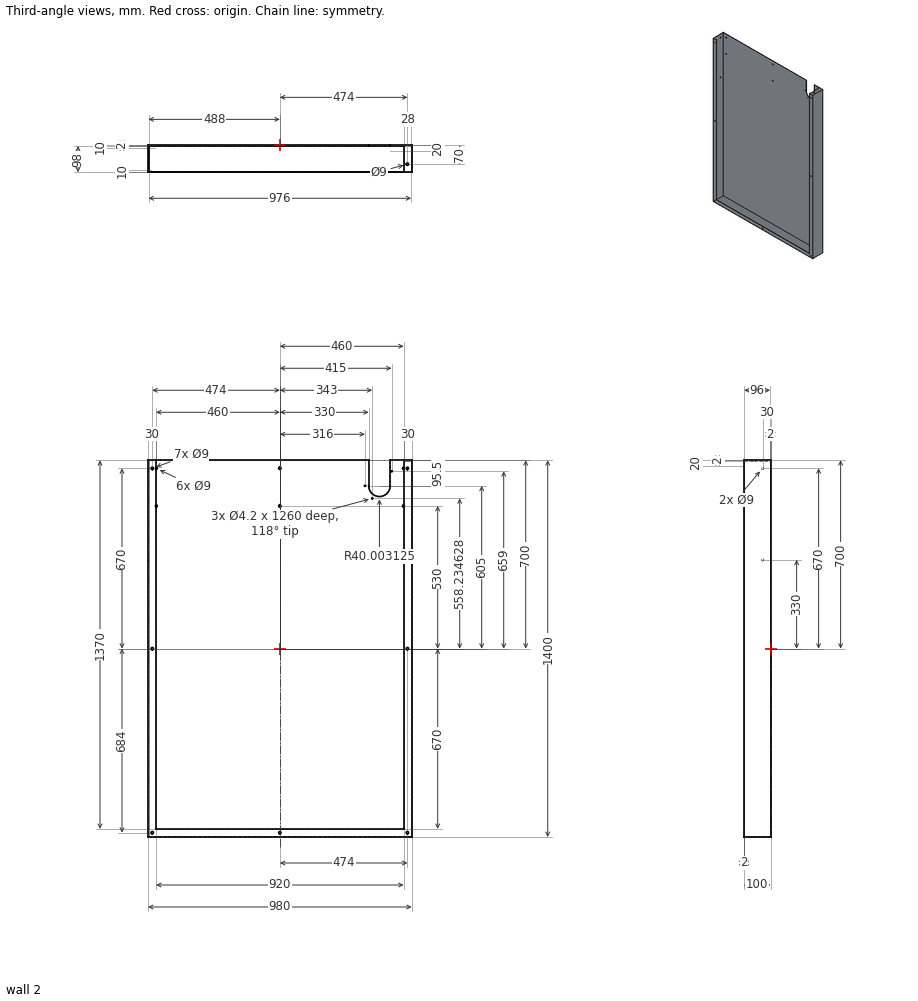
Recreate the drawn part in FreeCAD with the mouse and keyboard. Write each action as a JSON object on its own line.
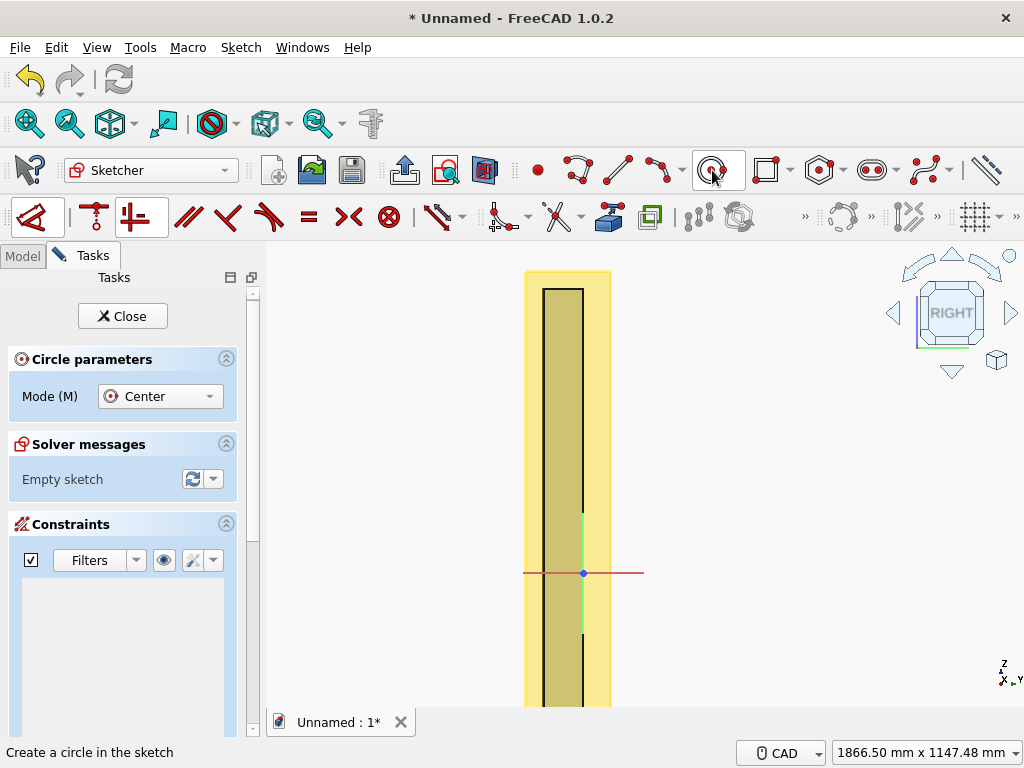
{"action": "scroll", "coordinate": [571, 301], "scroll_direction": "up", "scroll_amount": 13}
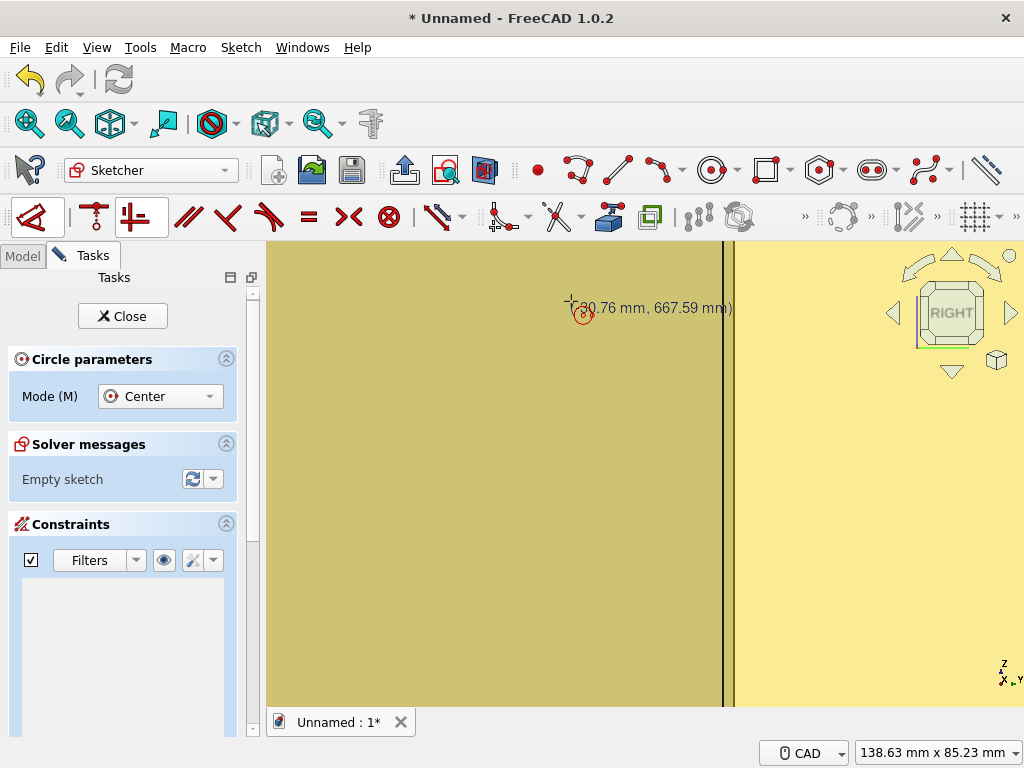
{"action": "scroll", "coordinate": [571, 342], "scroll_direction": "down", "scroll_amount": 13}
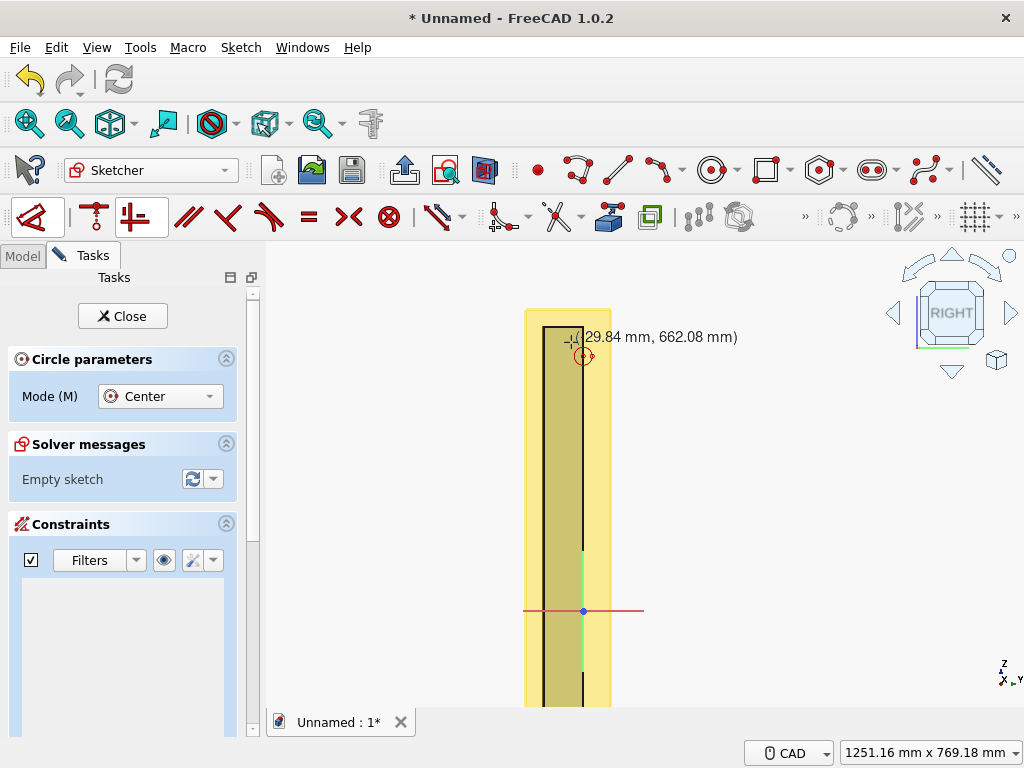
{"action": "scroll", "coordinate": [571, 339], "scroll_direction": "up", "scroll_amount": 2}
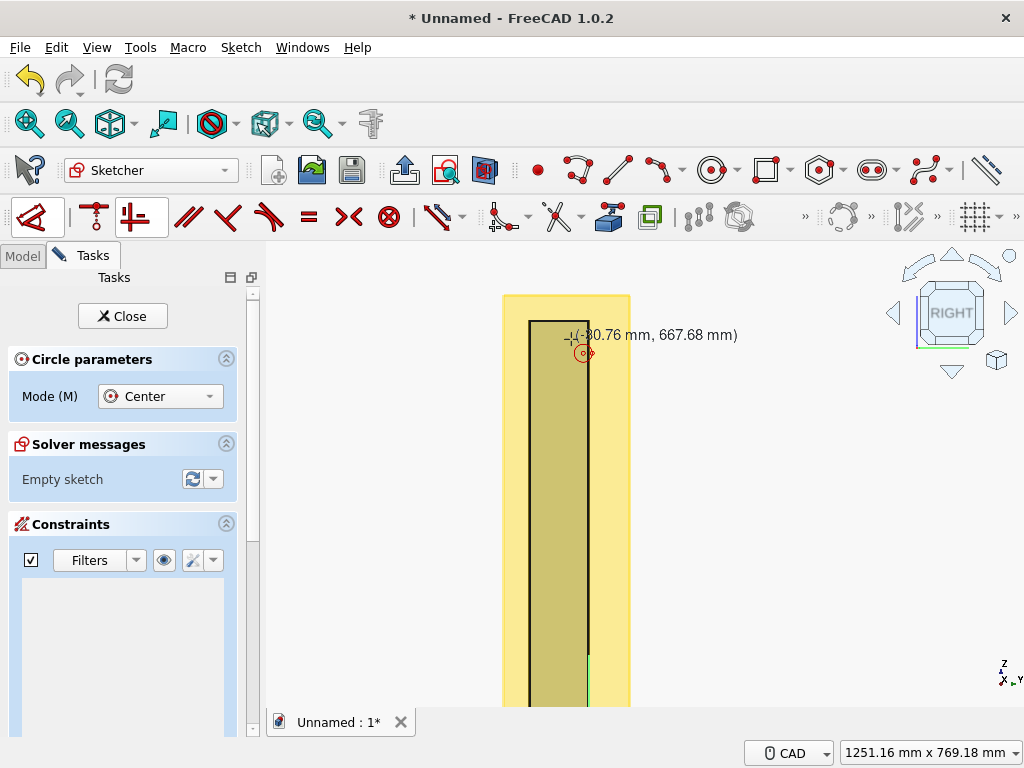
{"action": "left_click", "coordinate": [571, 339]}
{"action": "mouse_move", "coordinate": [573, 337]}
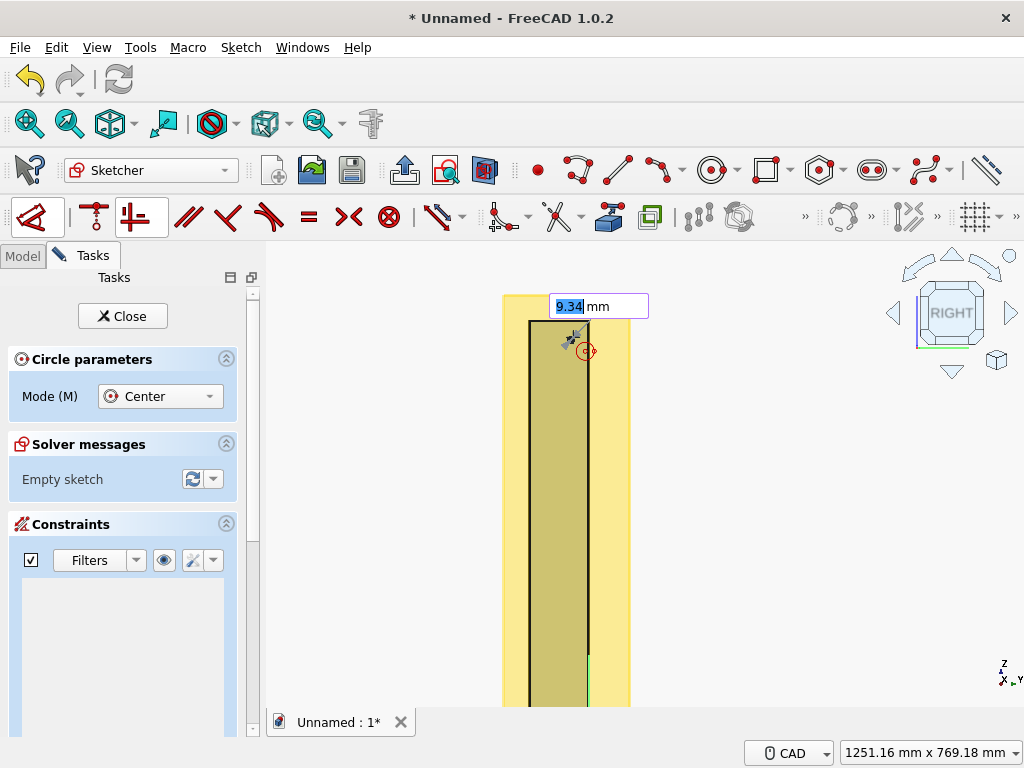
{"action": "type", "text": "9"}
{"action": "key", "text": "Return"}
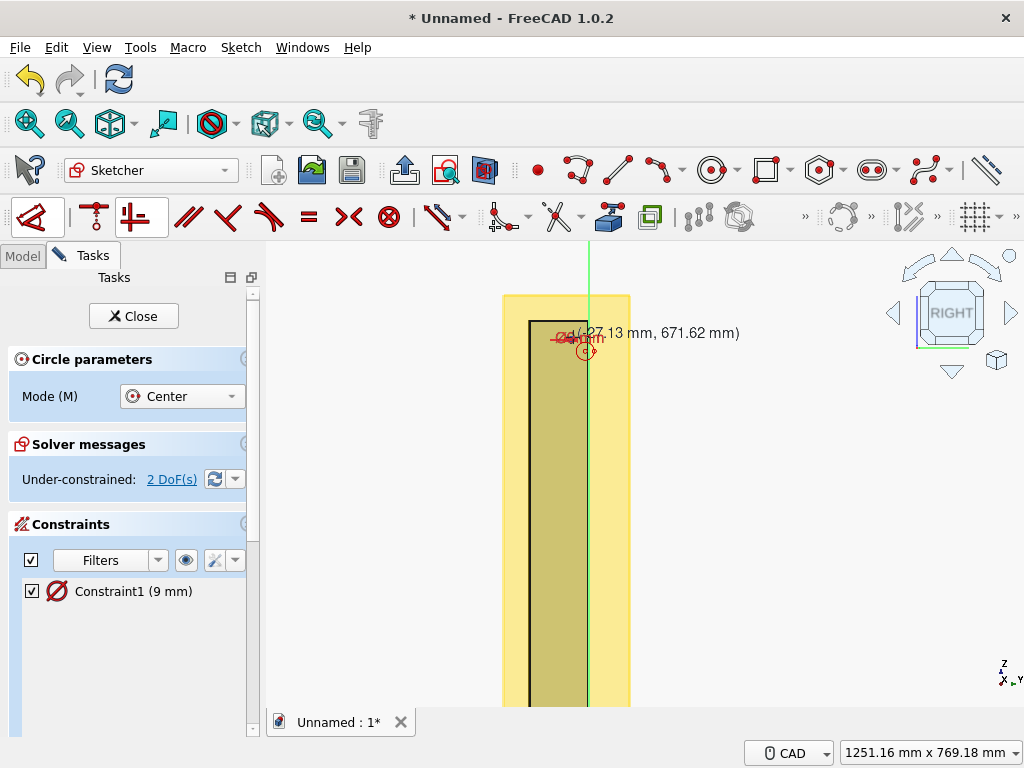
{"action": "scroll", "coordinate": [571, 545], "scroll_direction": "up", "scroll_amount": 11}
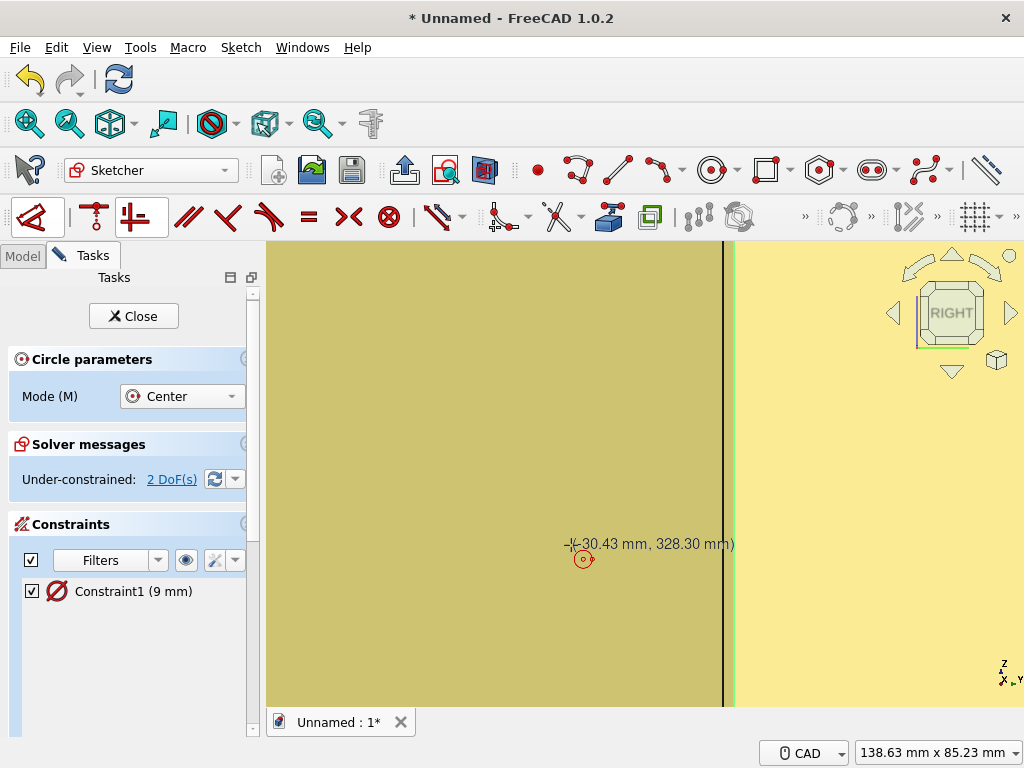
{"action": "scroll", "coordinate": [571, 472], "scroll_direction": "down", "scroll_amount": 13}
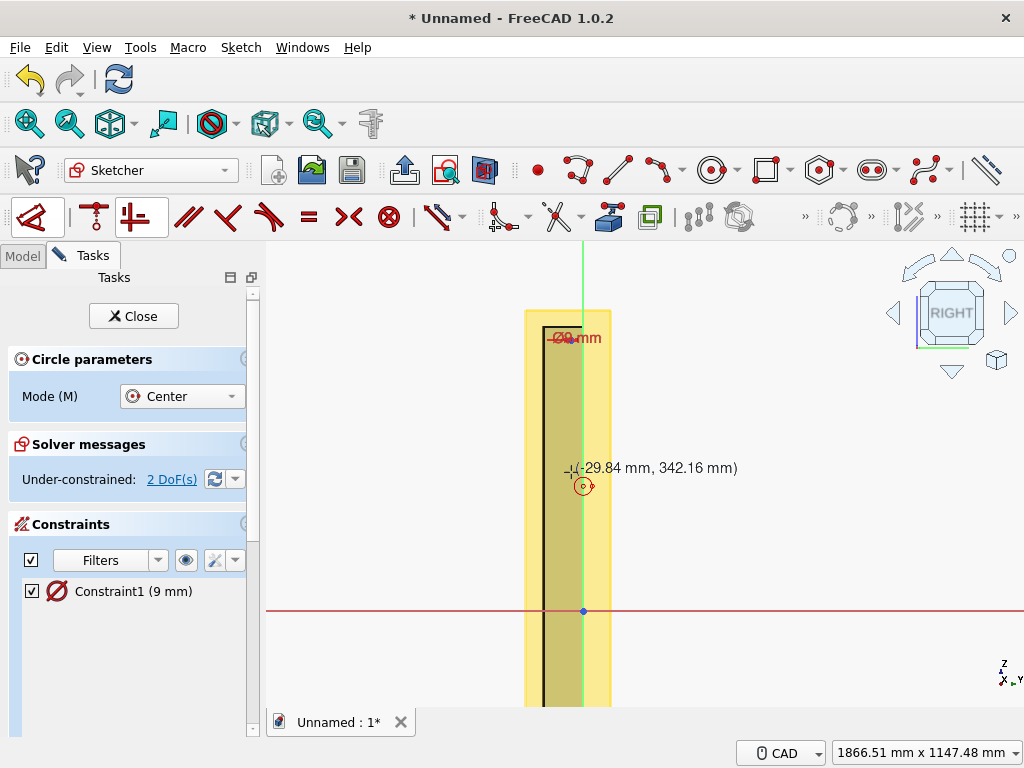
{"action": "scroll", "coordinate": [571, 477], "scroll_direction": "up", "scroll_amount": 2}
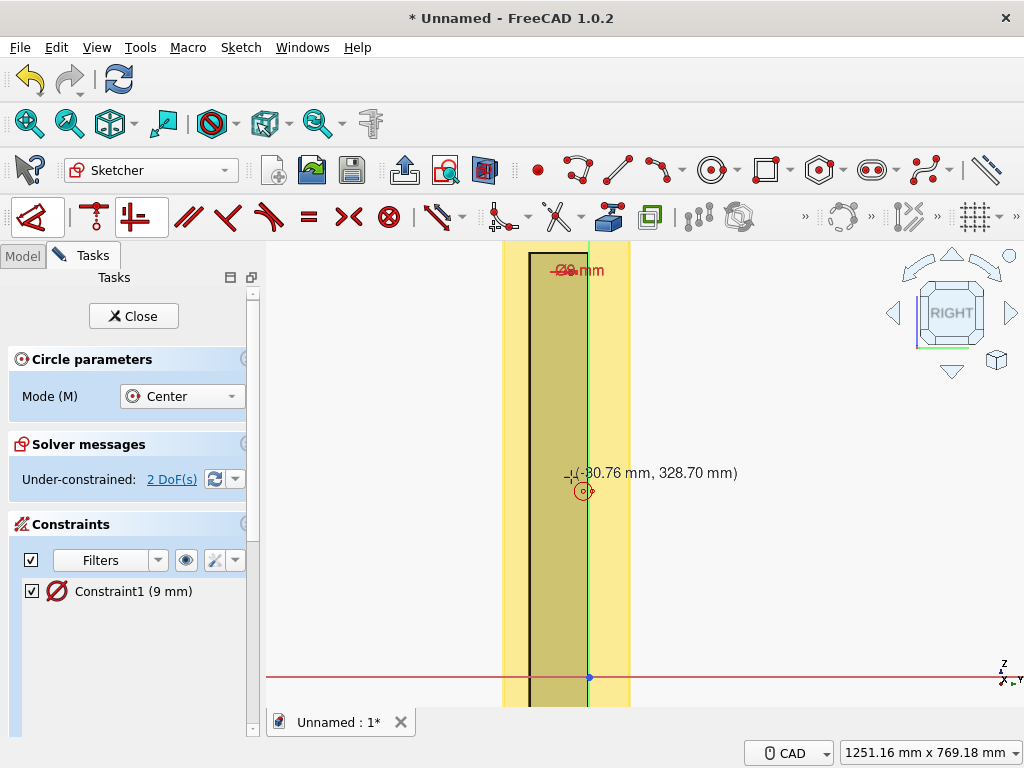
{"action": "left_click", "coordinate": [571, 477]}
{"action": "mouse_move", "coordinate": [573, 476]}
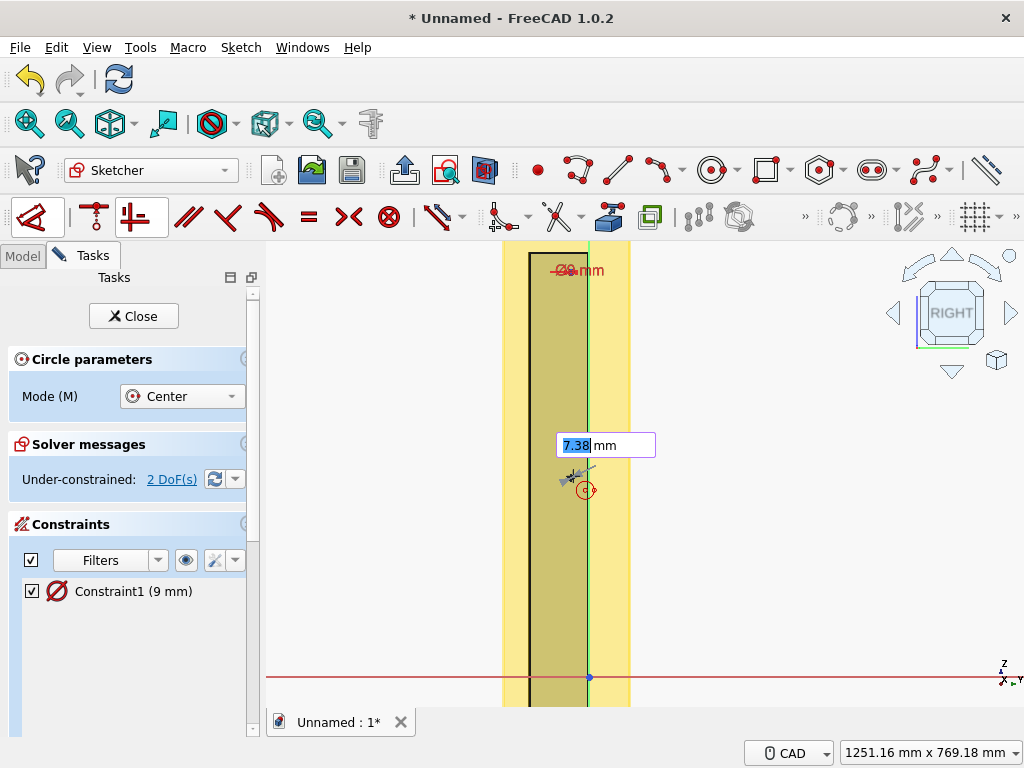
{"action": "type", "text": "9"}
{"action": "key", "text": "Return"}
{"action": "key", "text": "Escape"}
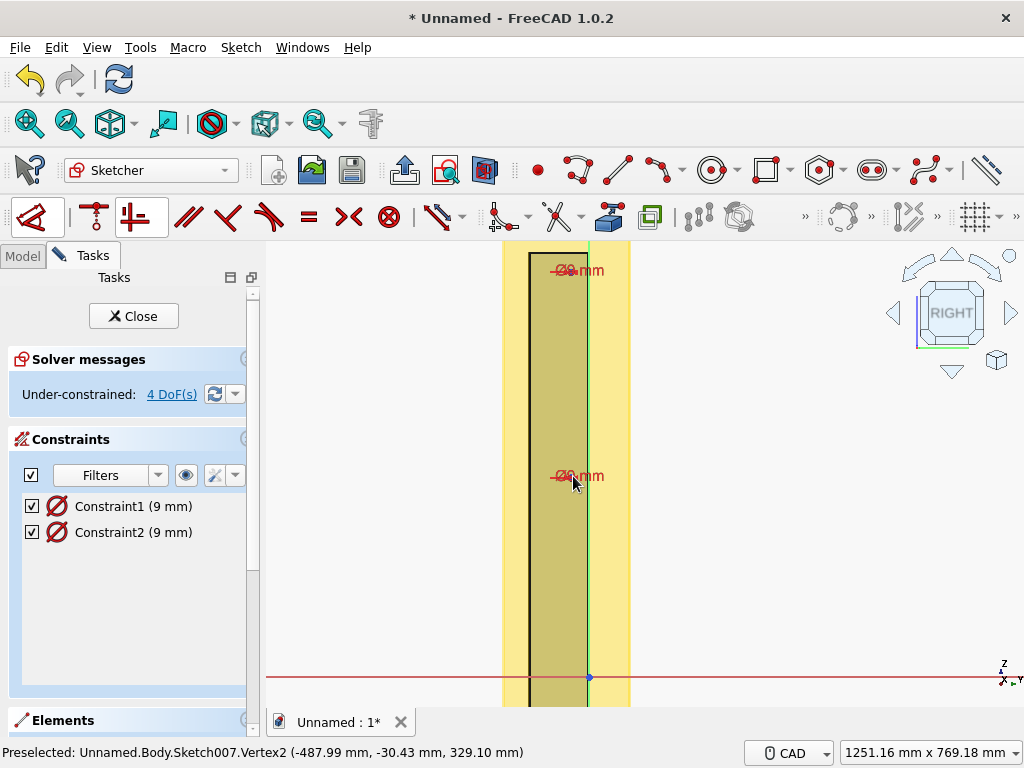
{"action": "scroll", "coordinate": [571, 272], "scroll_direction": "up", "scroll_amount": 4}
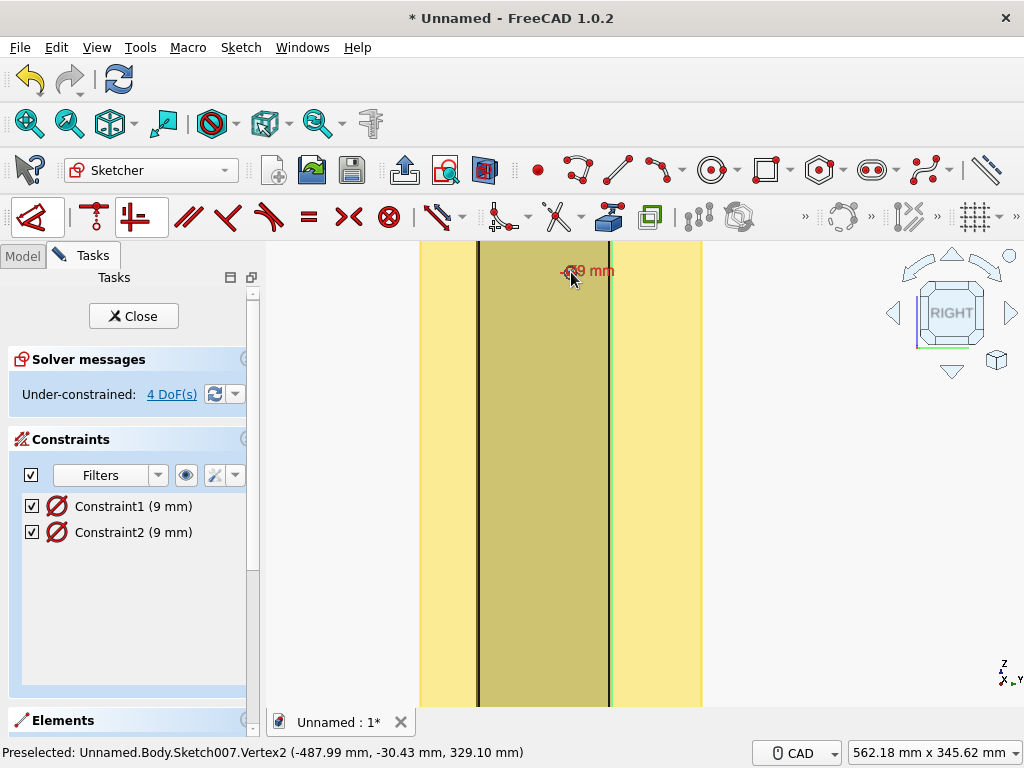
{"action": "left_click", "coordinate": [571, 273]}